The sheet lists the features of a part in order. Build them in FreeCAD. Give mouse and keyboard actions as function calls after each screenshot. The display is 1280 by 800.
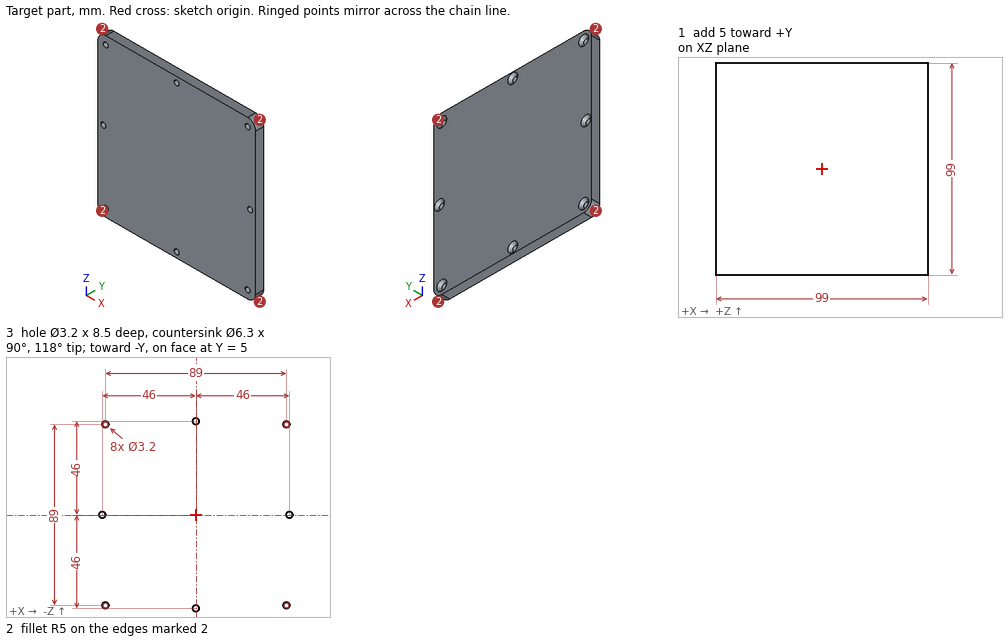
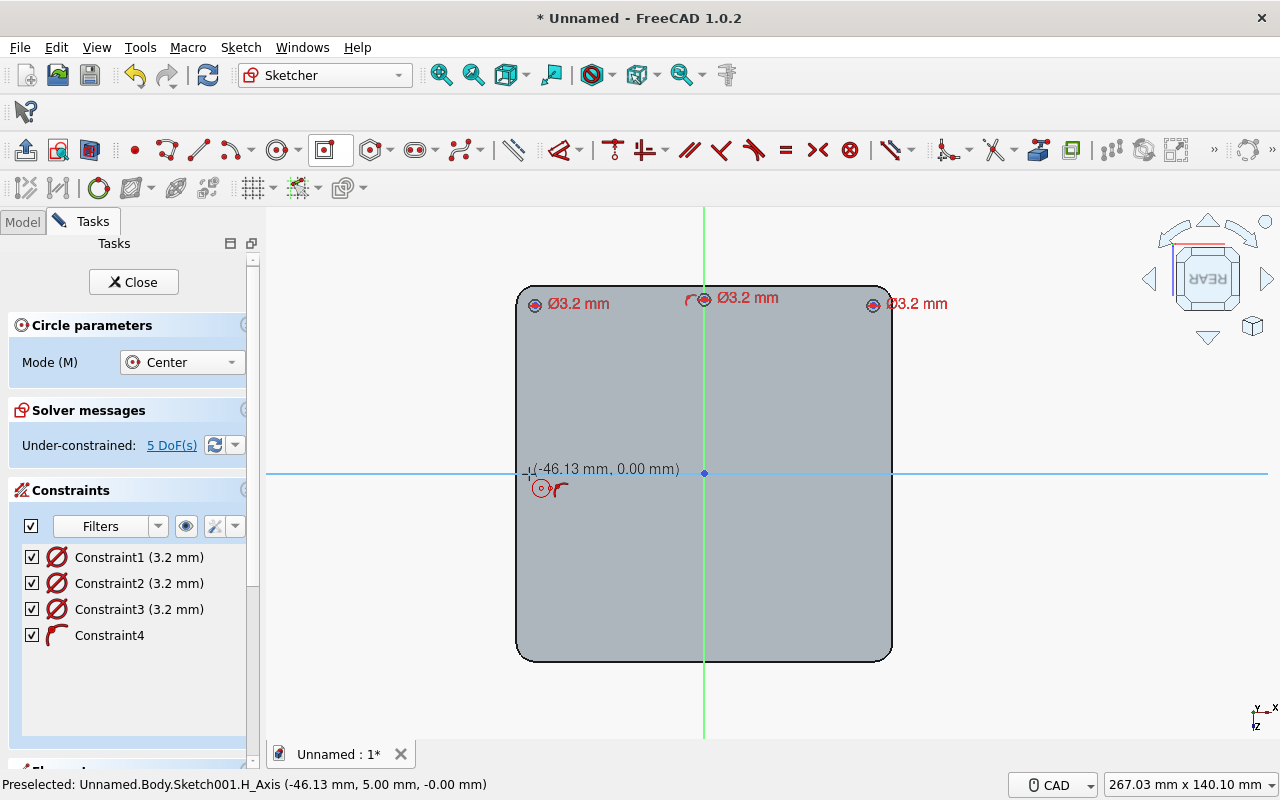
click(530, 474)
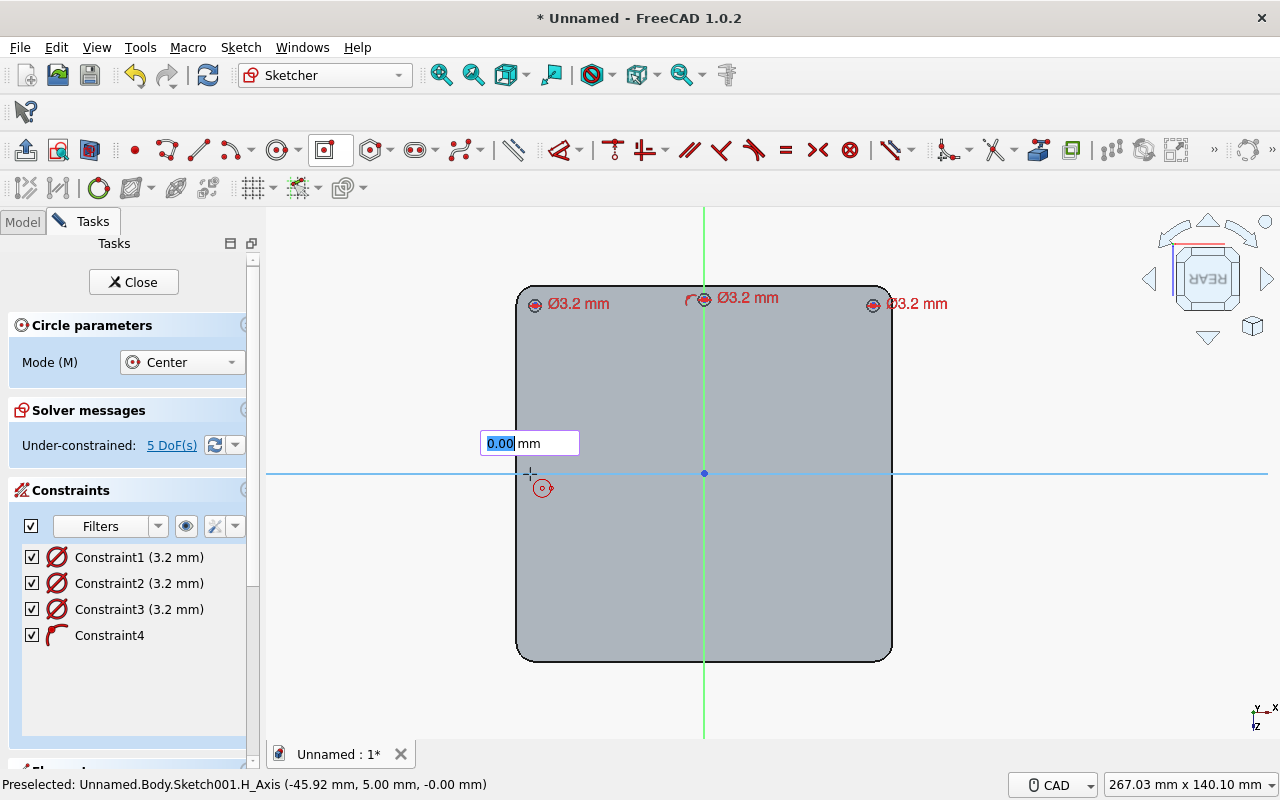
scroll(528, 479, up, 6)
move(526, 479)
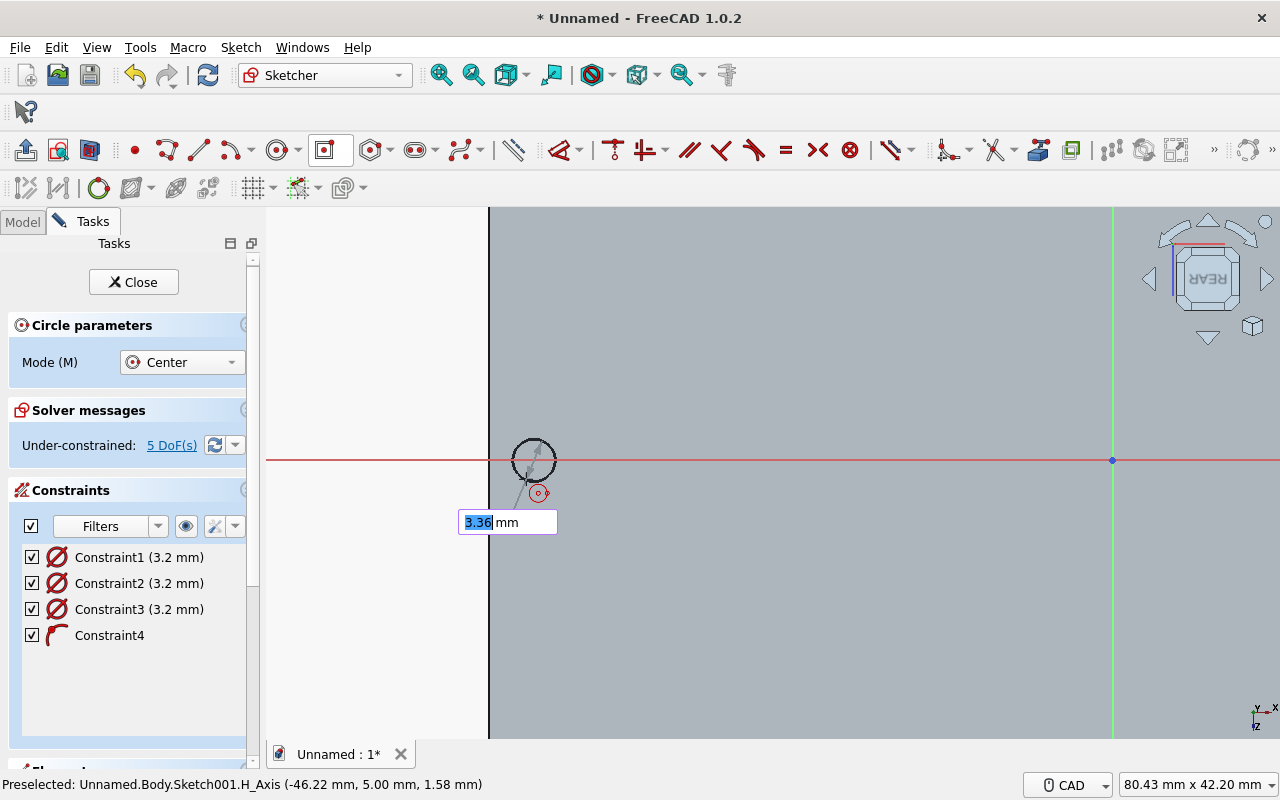
text(3.2)
key(Return)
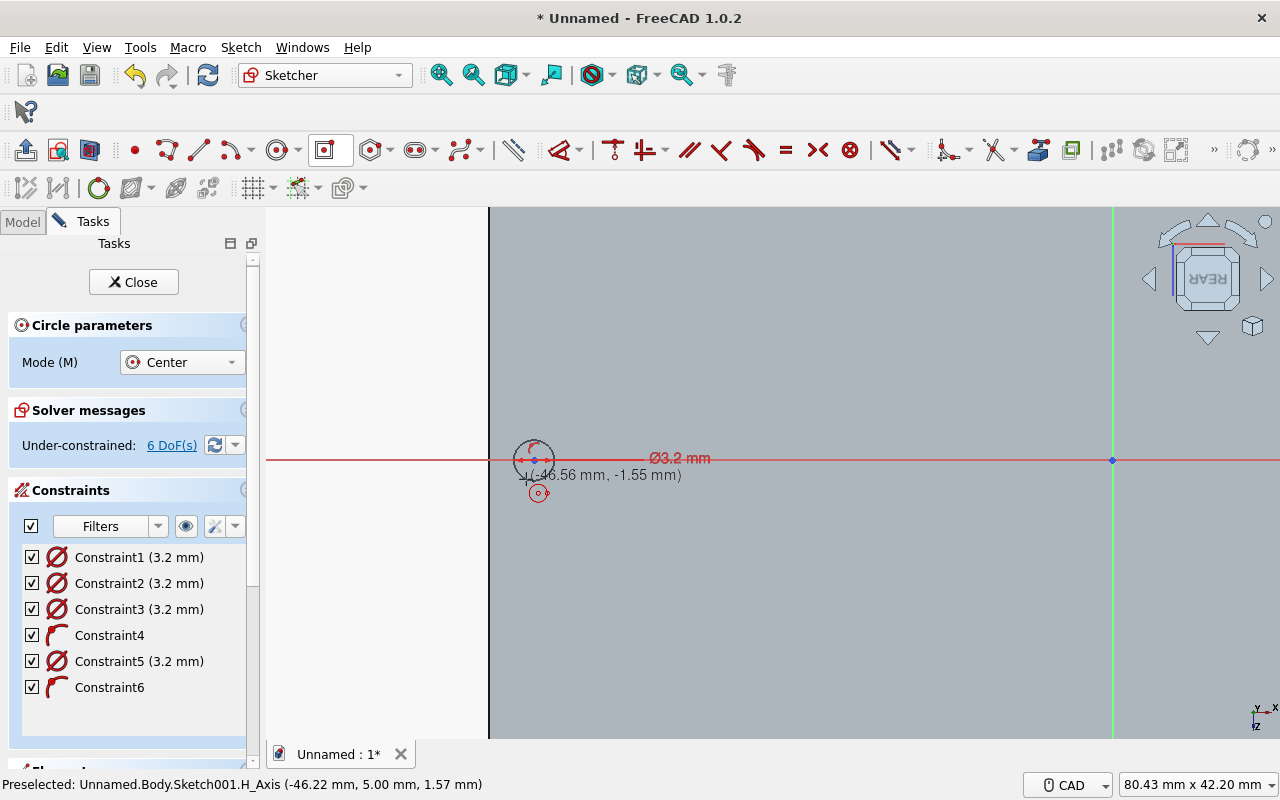
scroll(528, 478, down, 6)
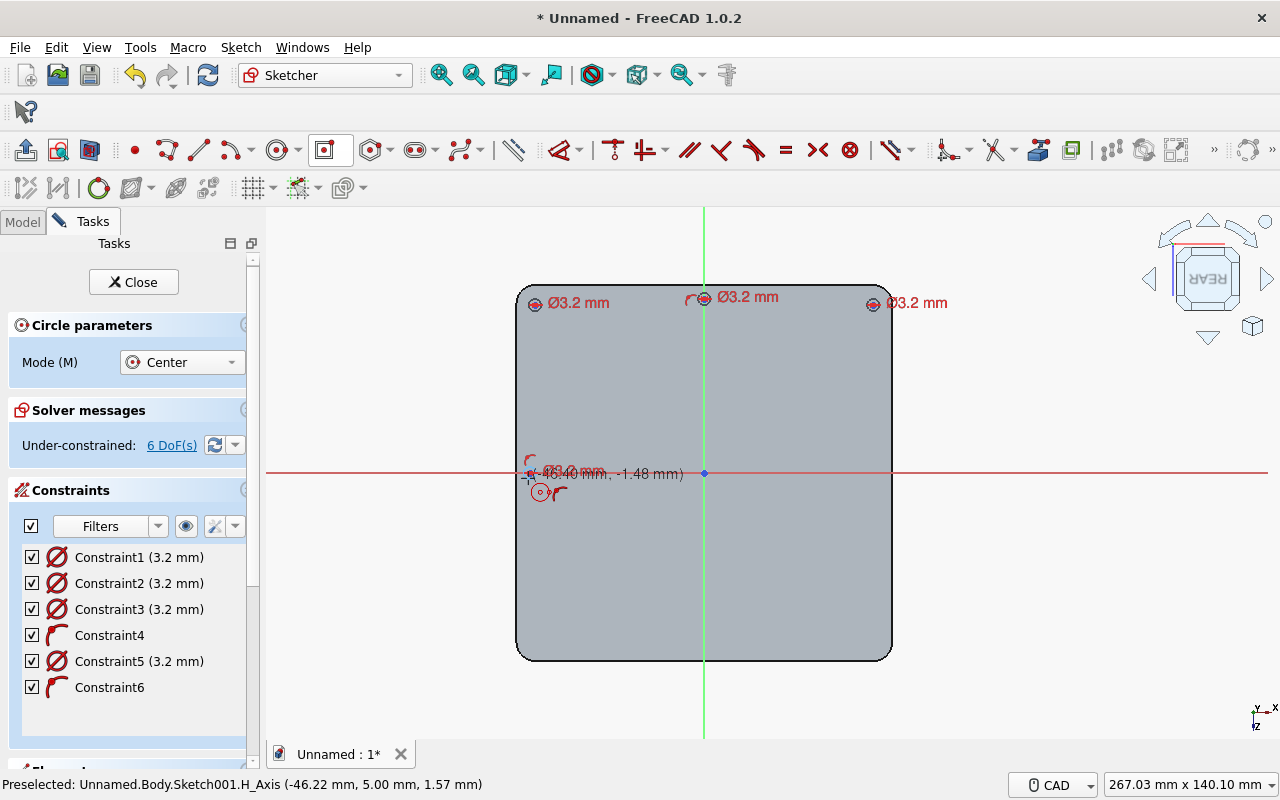
scroll(535, 642, up, 7)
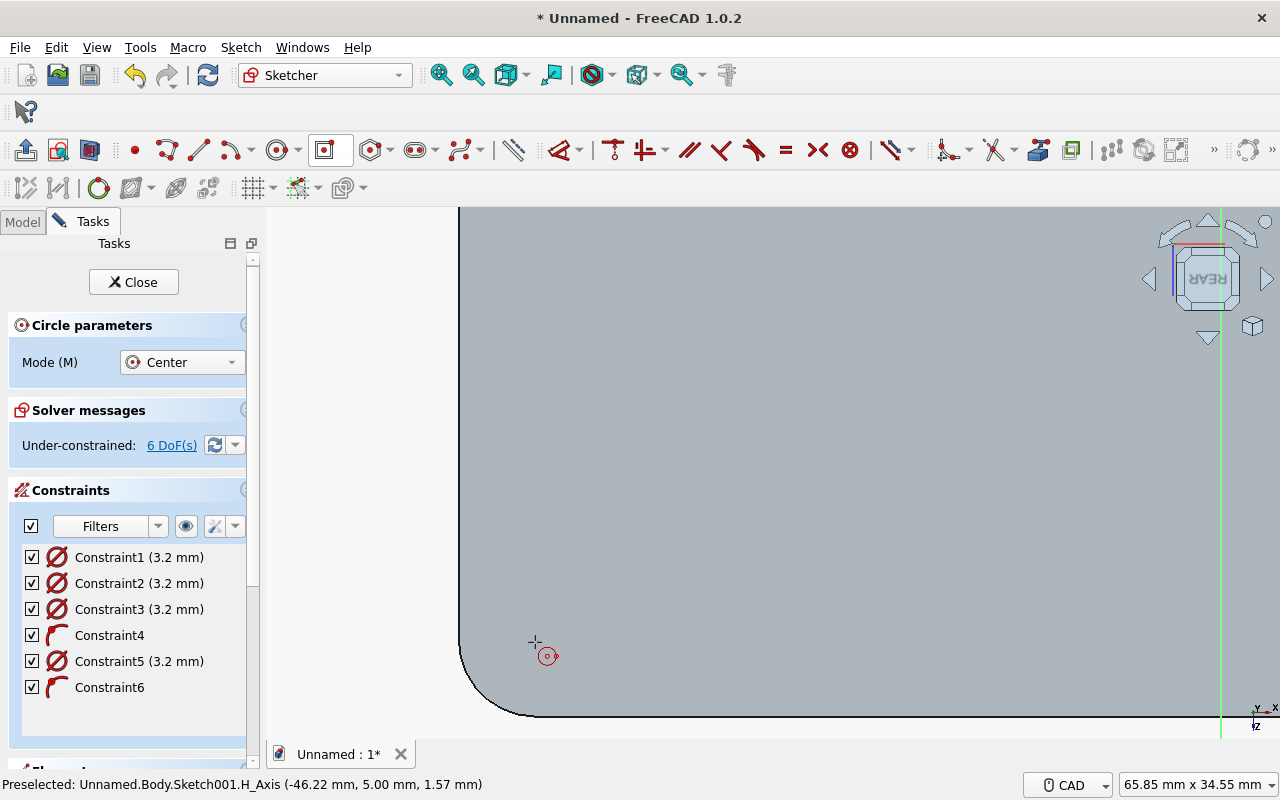
scroll(535, 643, down, 7)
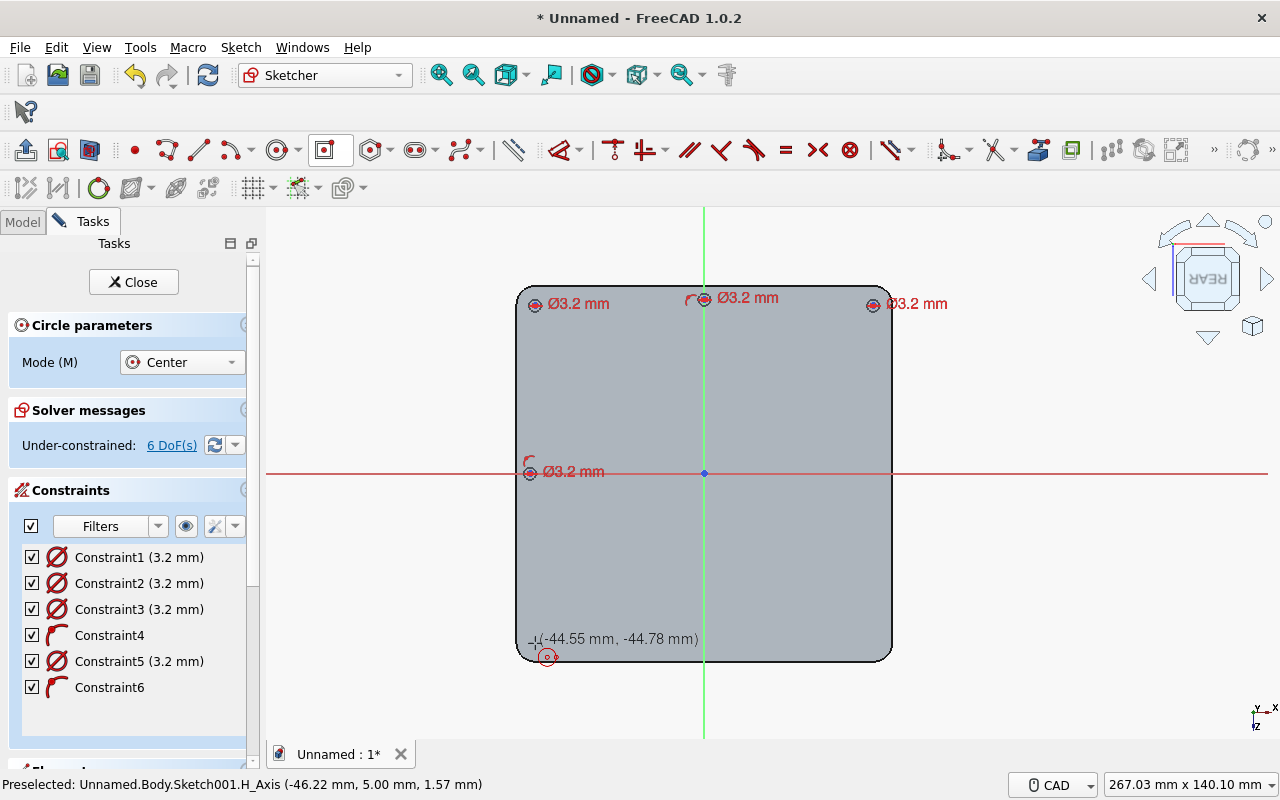
click(535, 643)
move(540, 638)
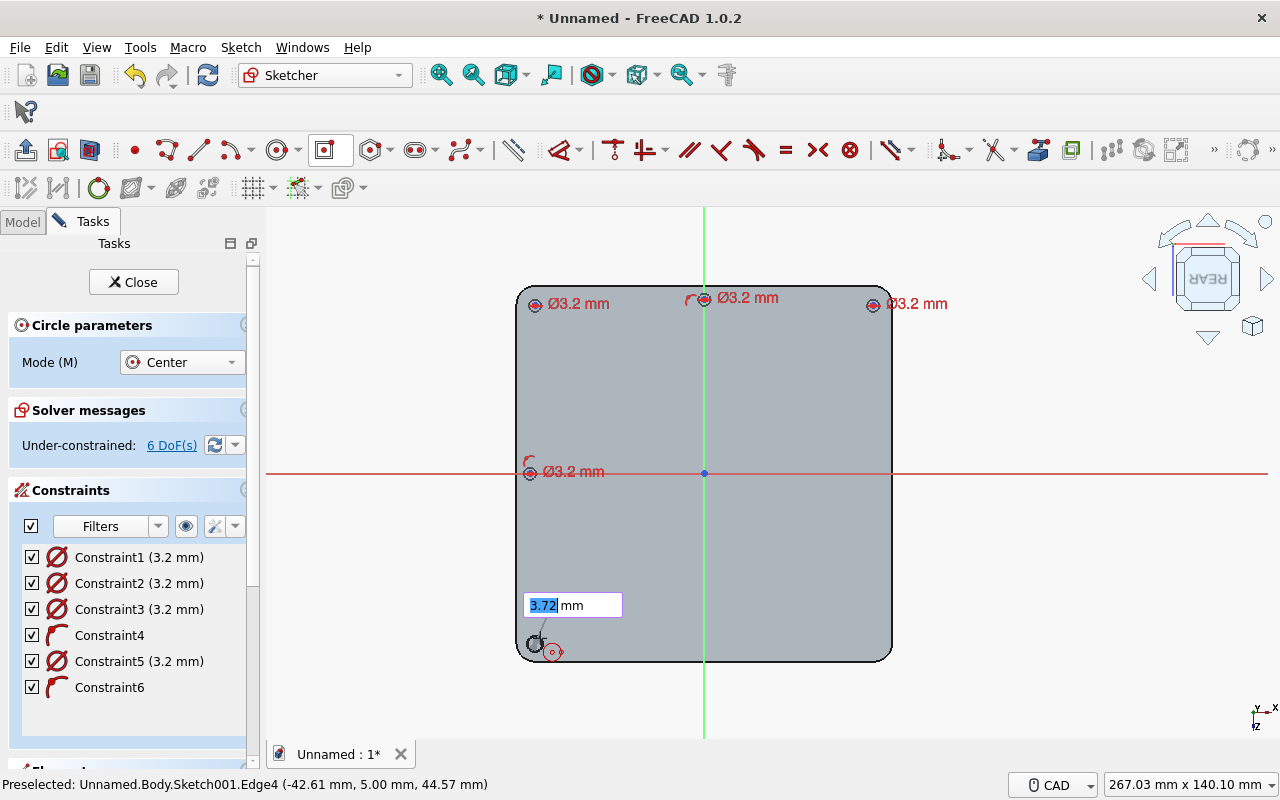
text(3.2)
key(Return)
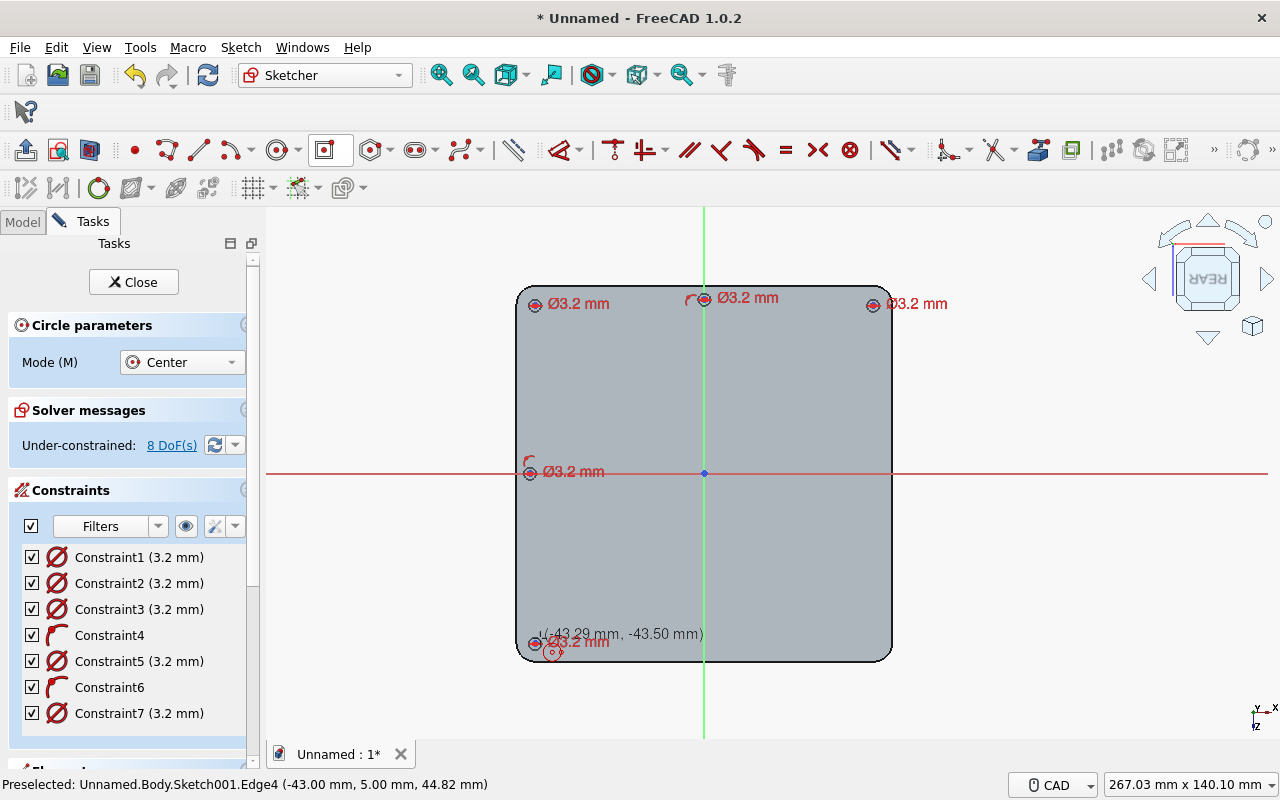
scroll(704, 648, up, 7)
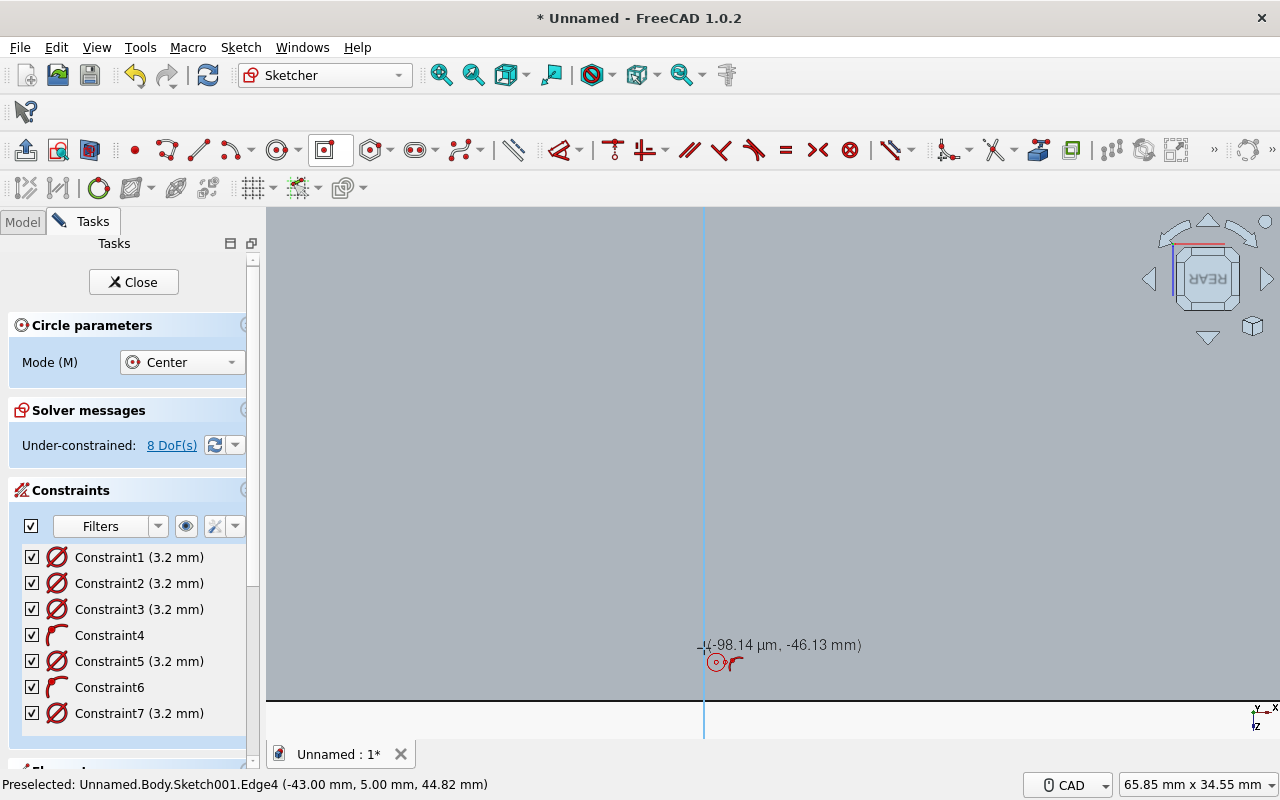
scroll(705, 648, down, 7)